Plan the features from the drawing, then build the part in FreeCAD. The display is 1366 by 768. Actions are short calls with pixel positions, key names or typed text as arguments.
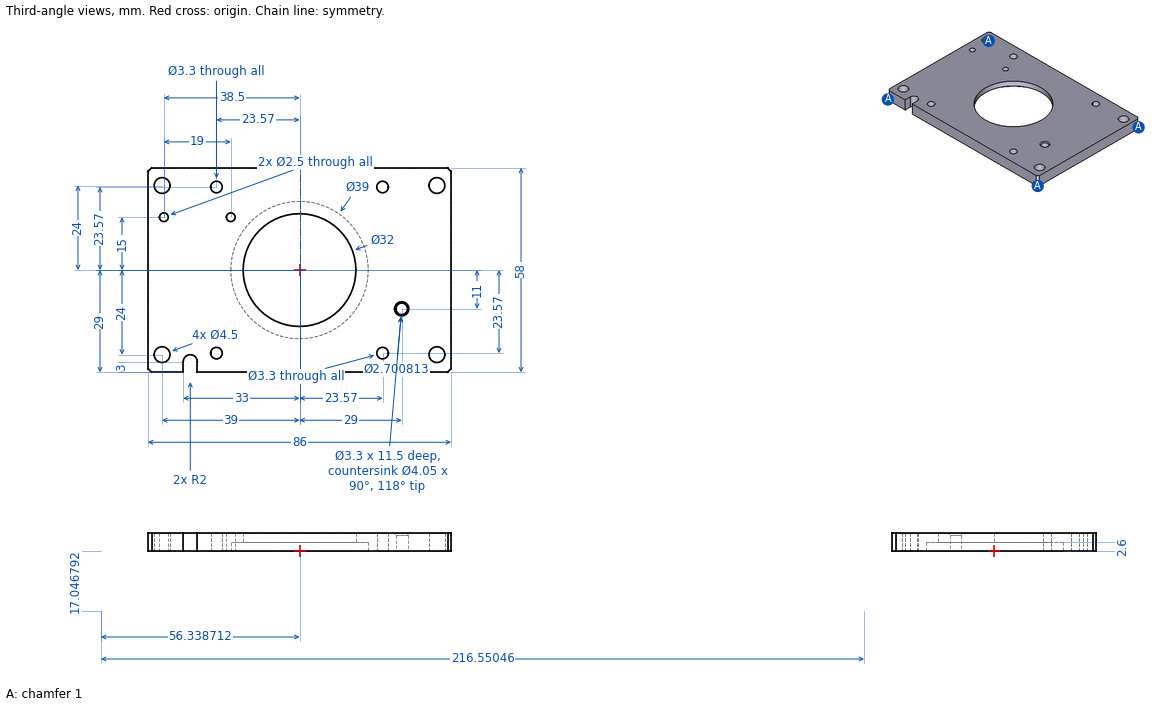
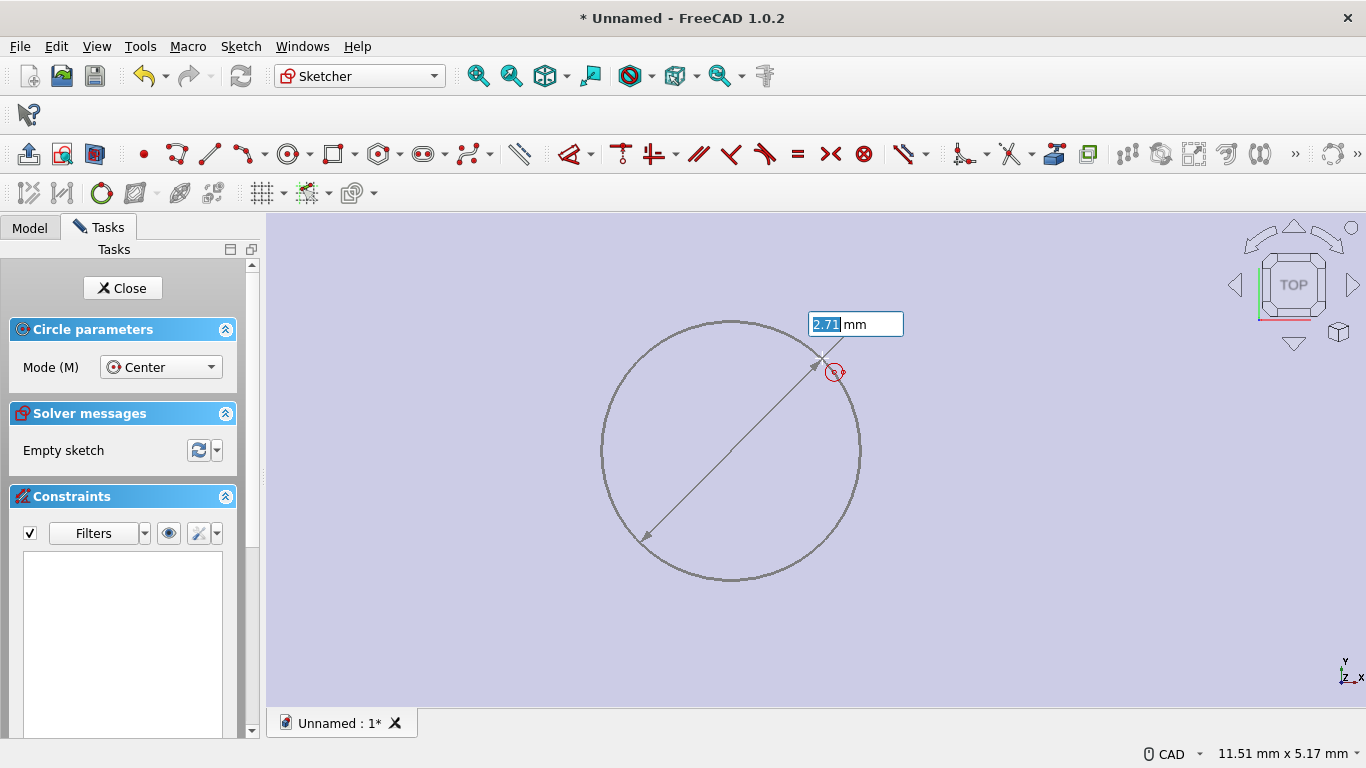
text(2.700813)
key(Return)
key(Escape)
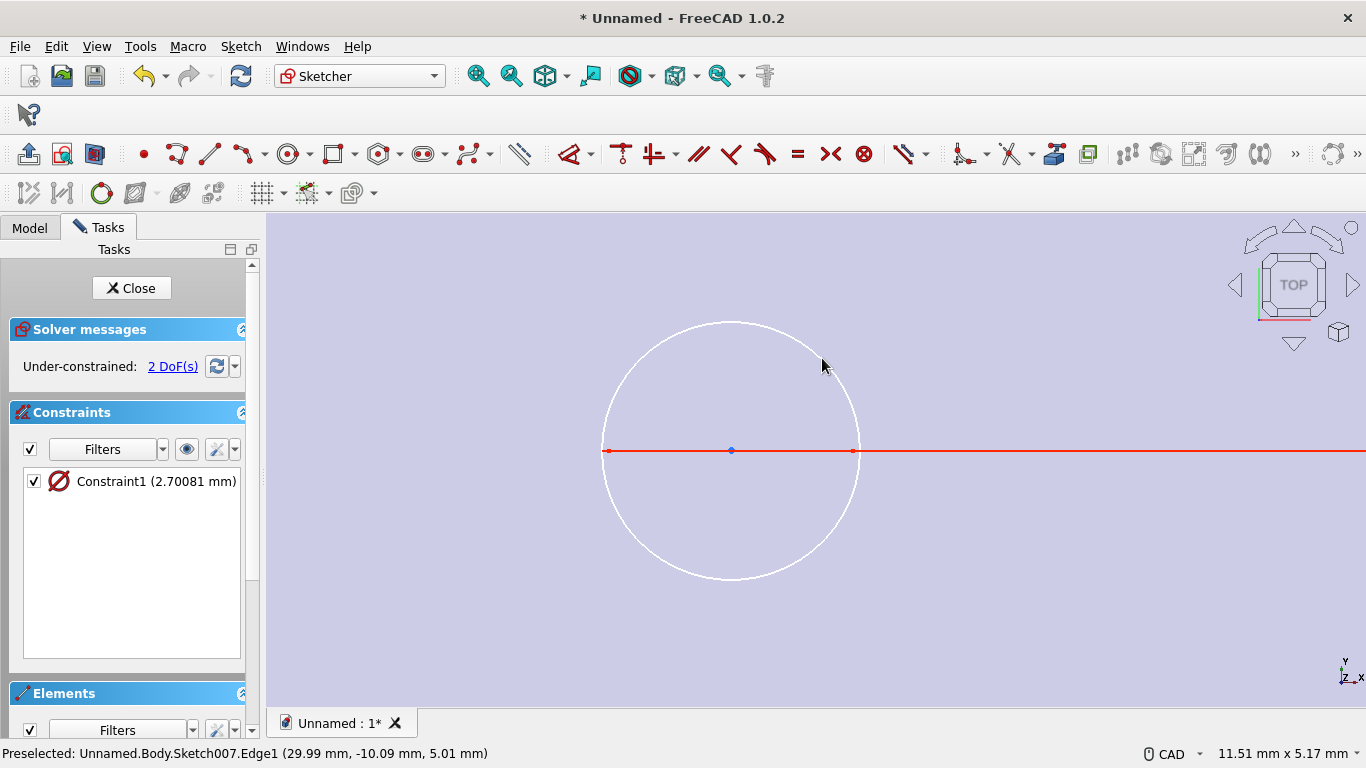
click(568, 154)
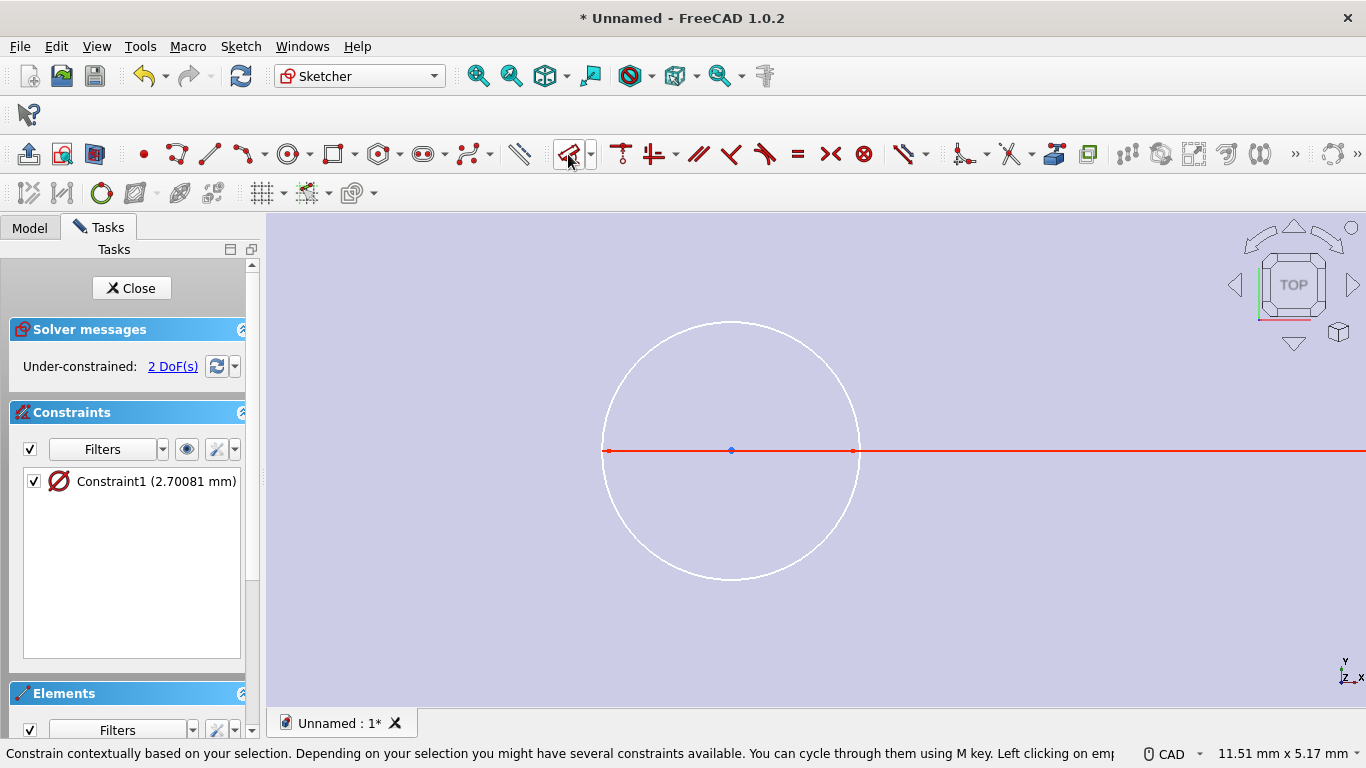
click(731, 451)
click(513, 485)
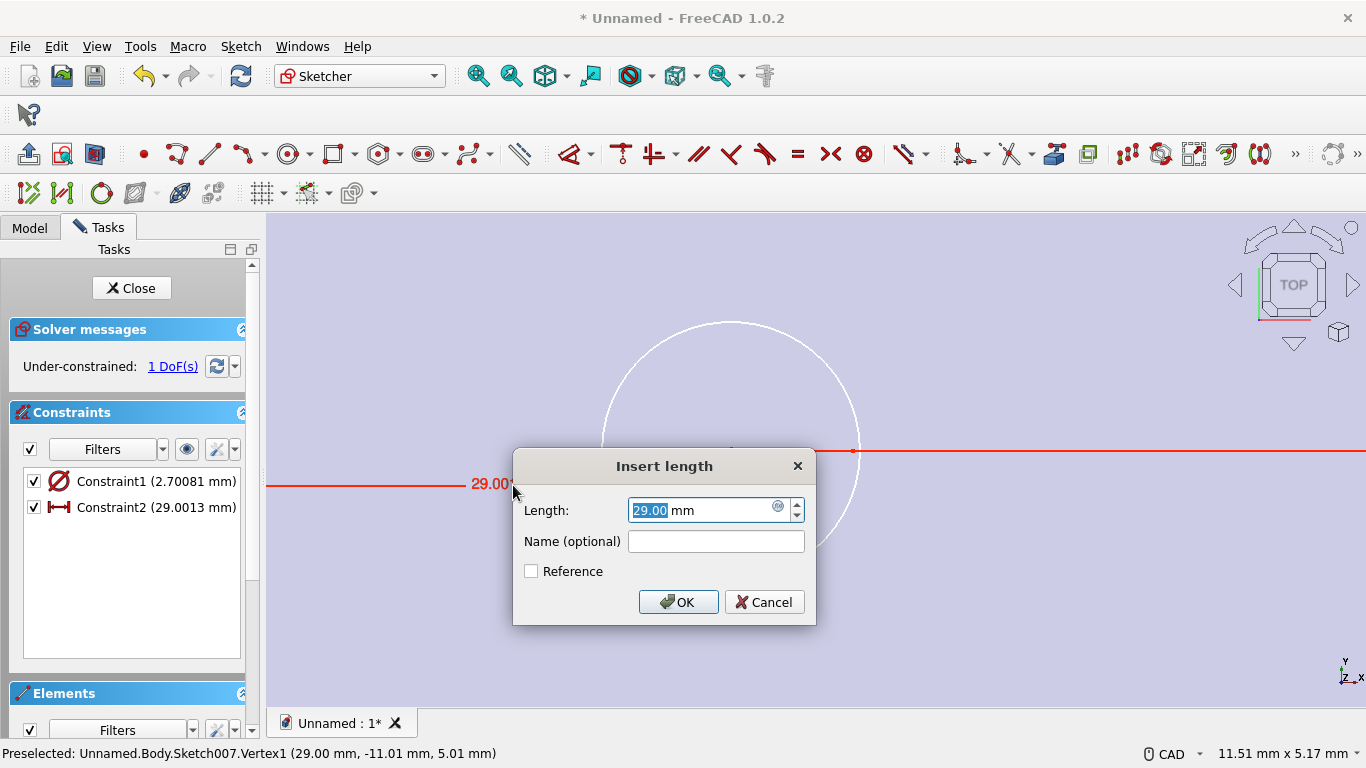
text(29)
key(Return)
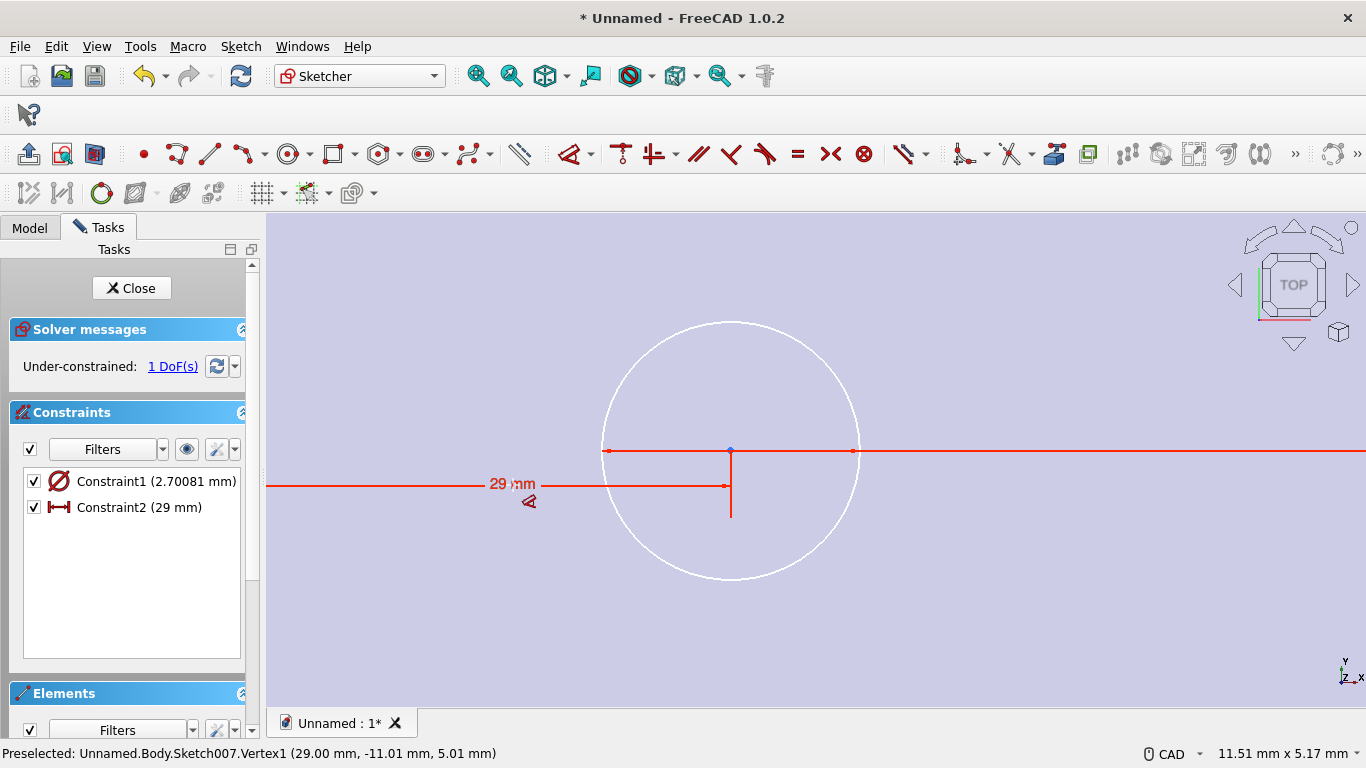
click(731, 451)
click(765, 346)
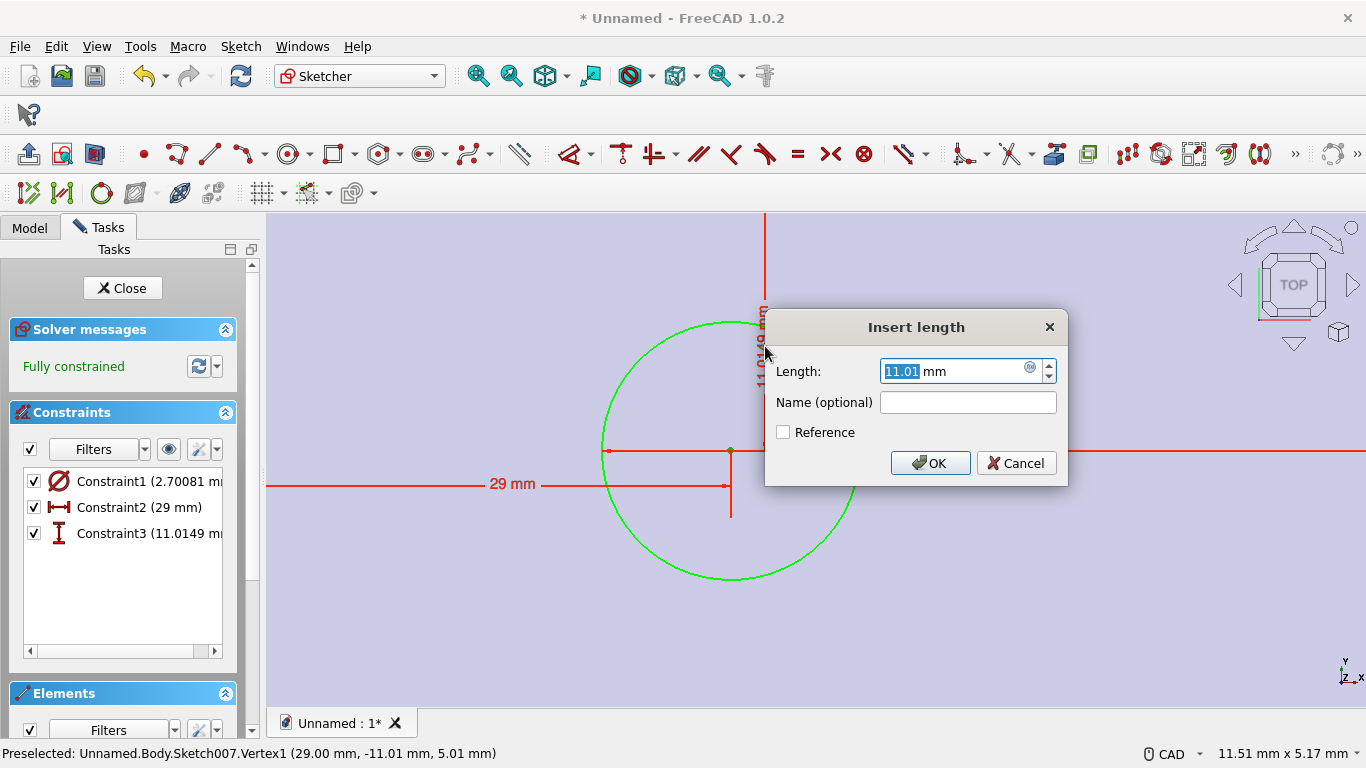
text(11)
key(Return)
key(Escape)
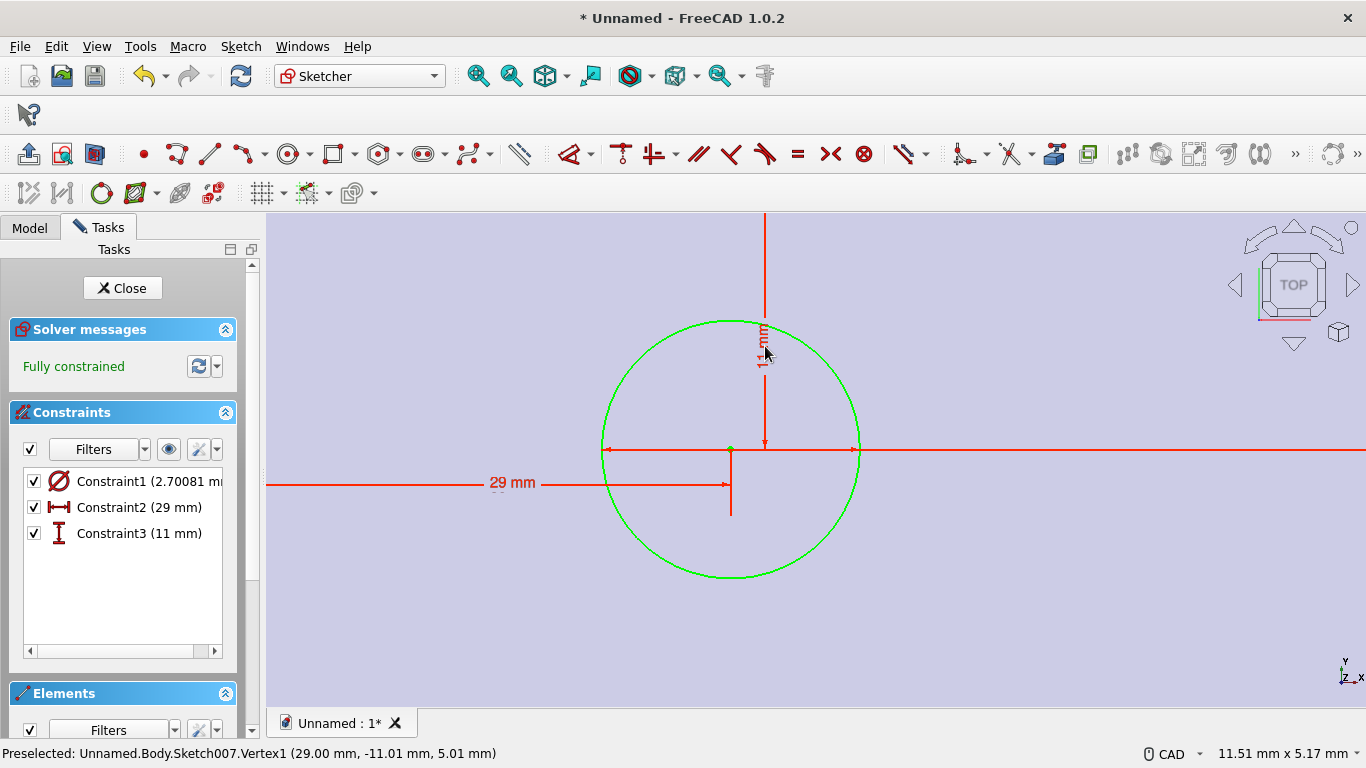
click(123, 288)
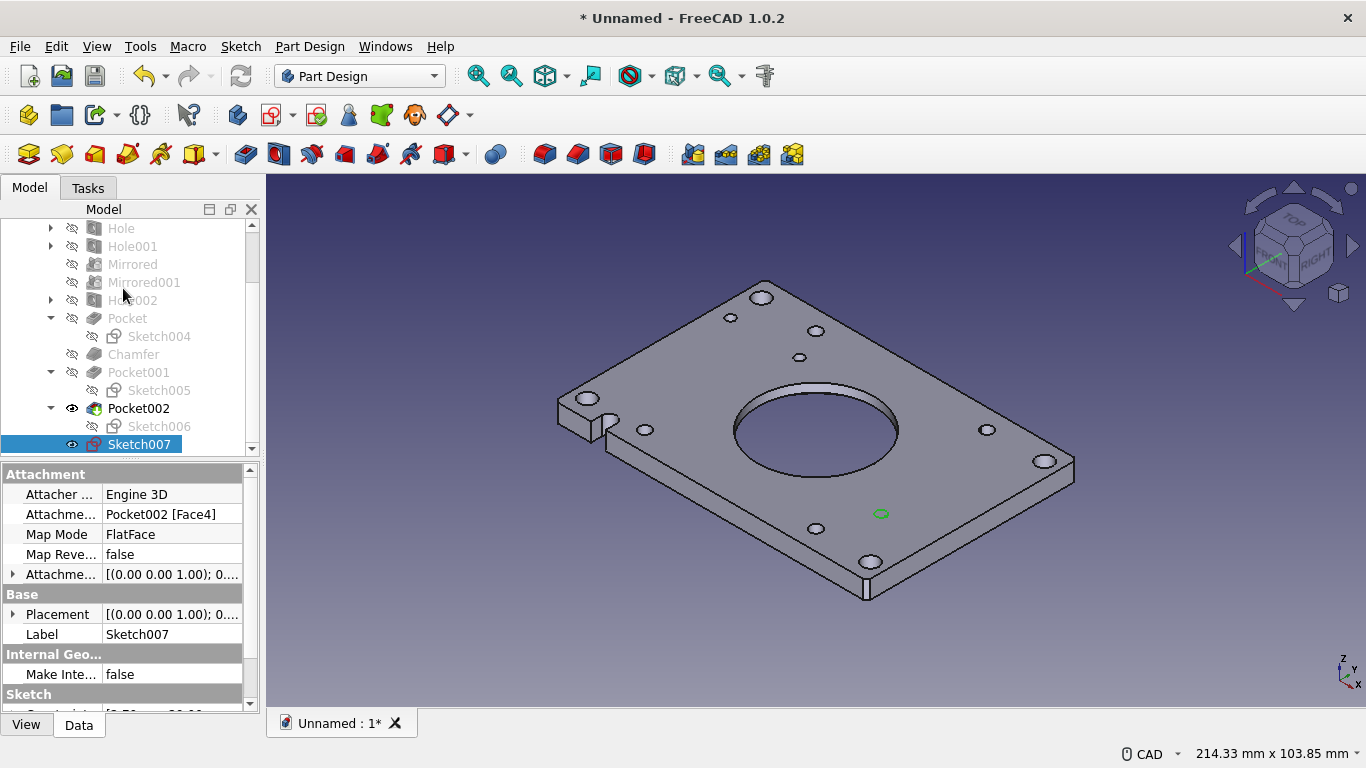
click(246, 154)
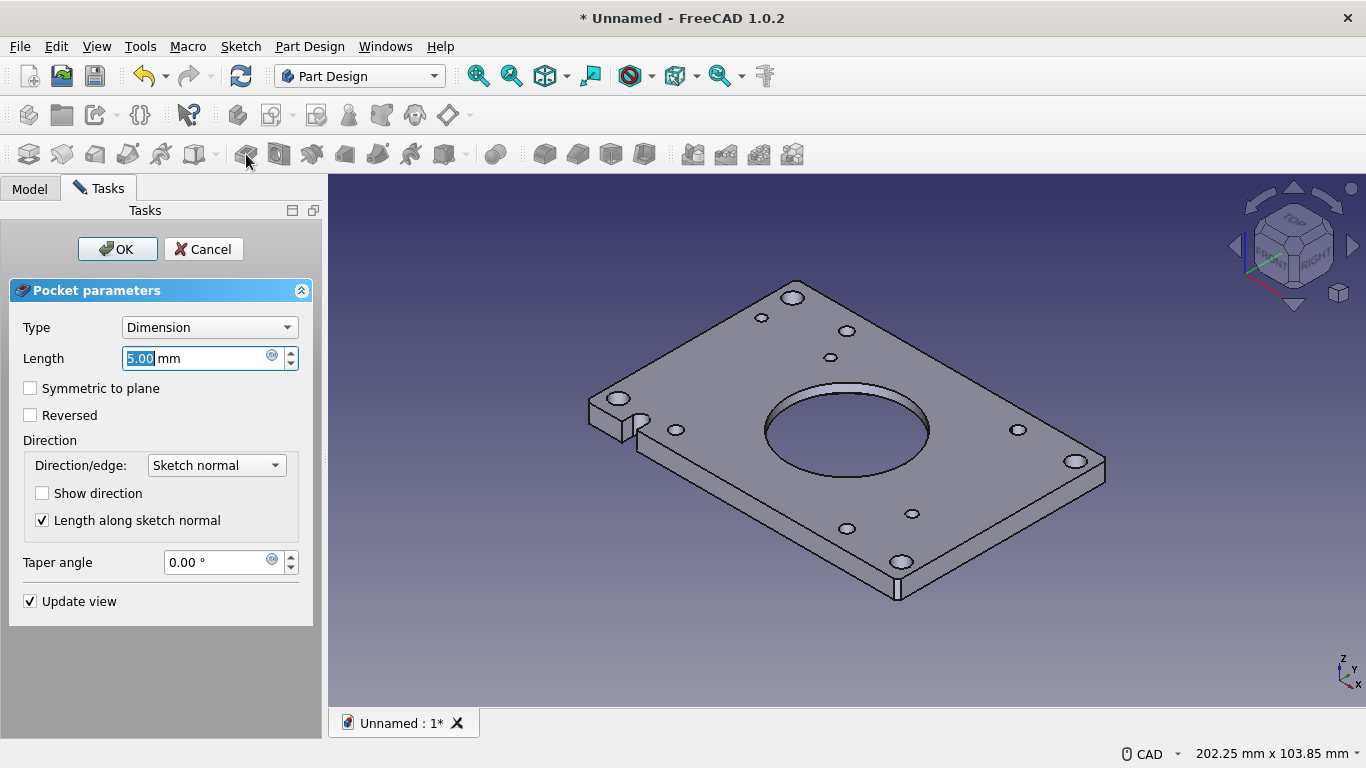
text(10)
key(Tab)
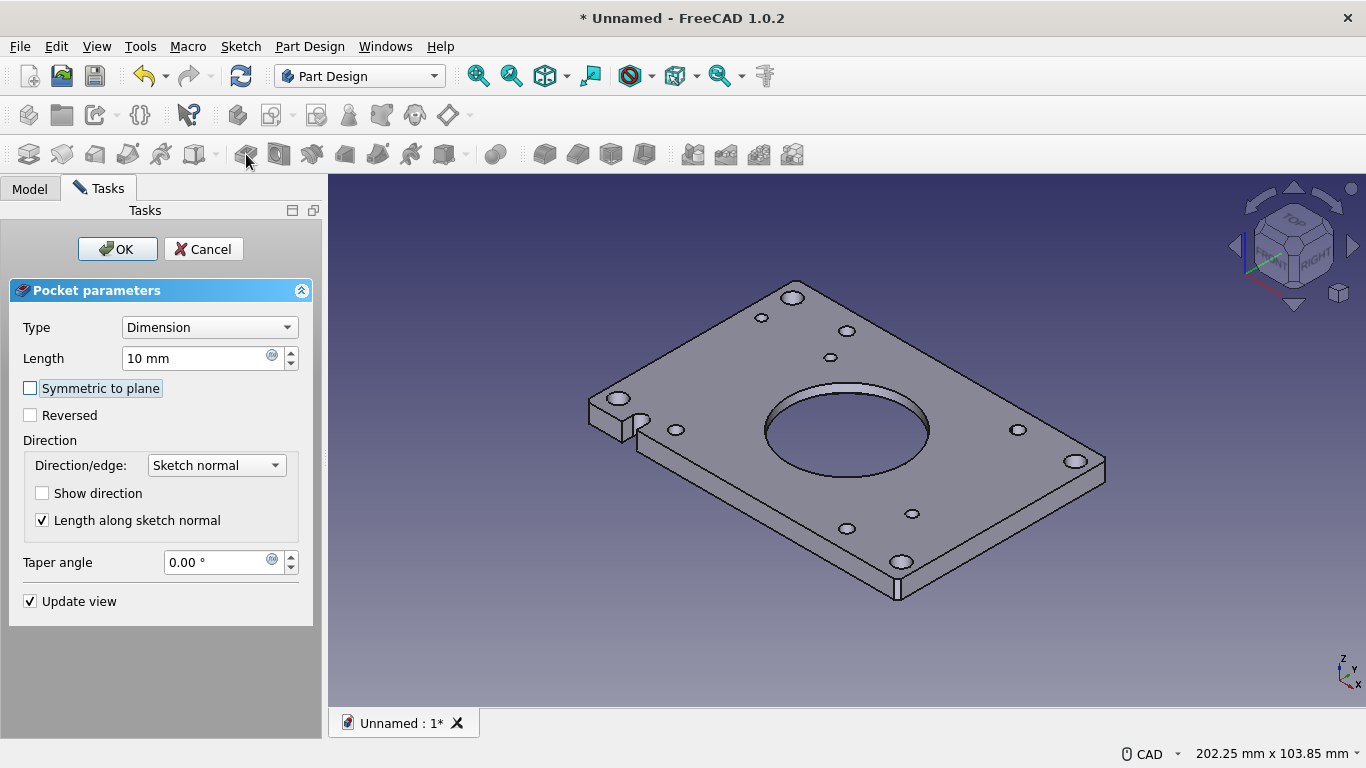
click(118, 249)